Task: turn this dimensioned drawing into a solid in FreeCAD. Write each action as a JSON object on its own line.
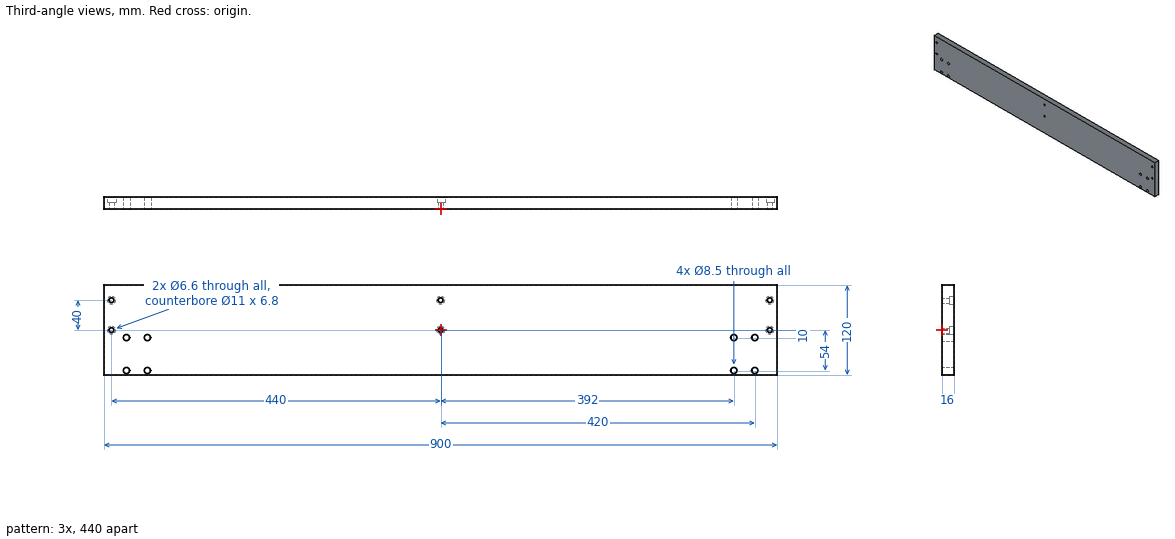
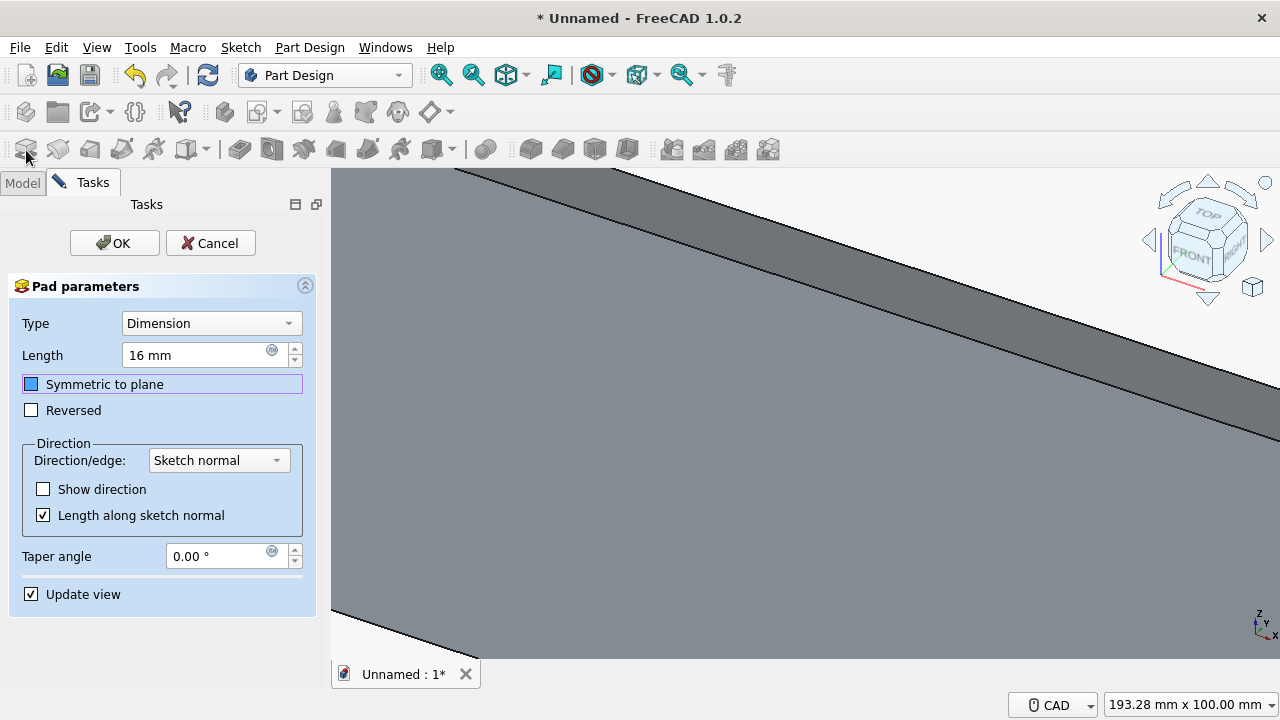
{"action": "left_click", "coordinate": [30, 410]}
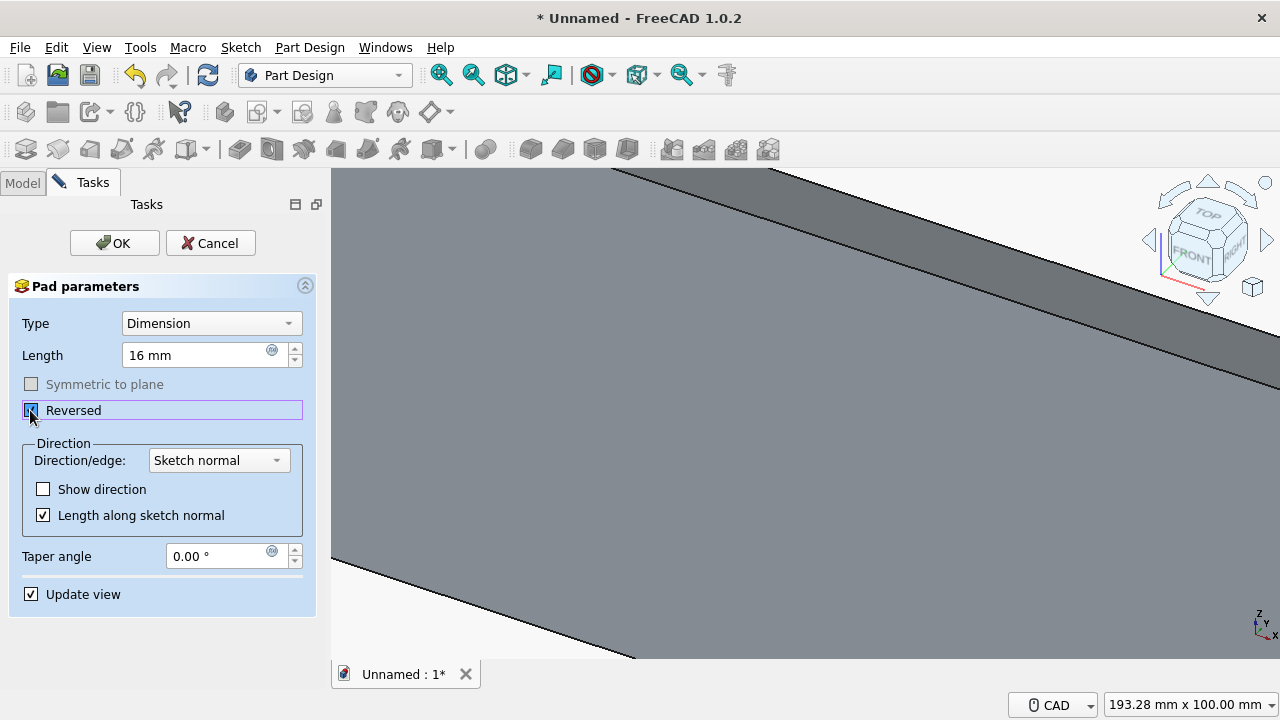
{"action": "left_click", "coordinate": [115, 243]}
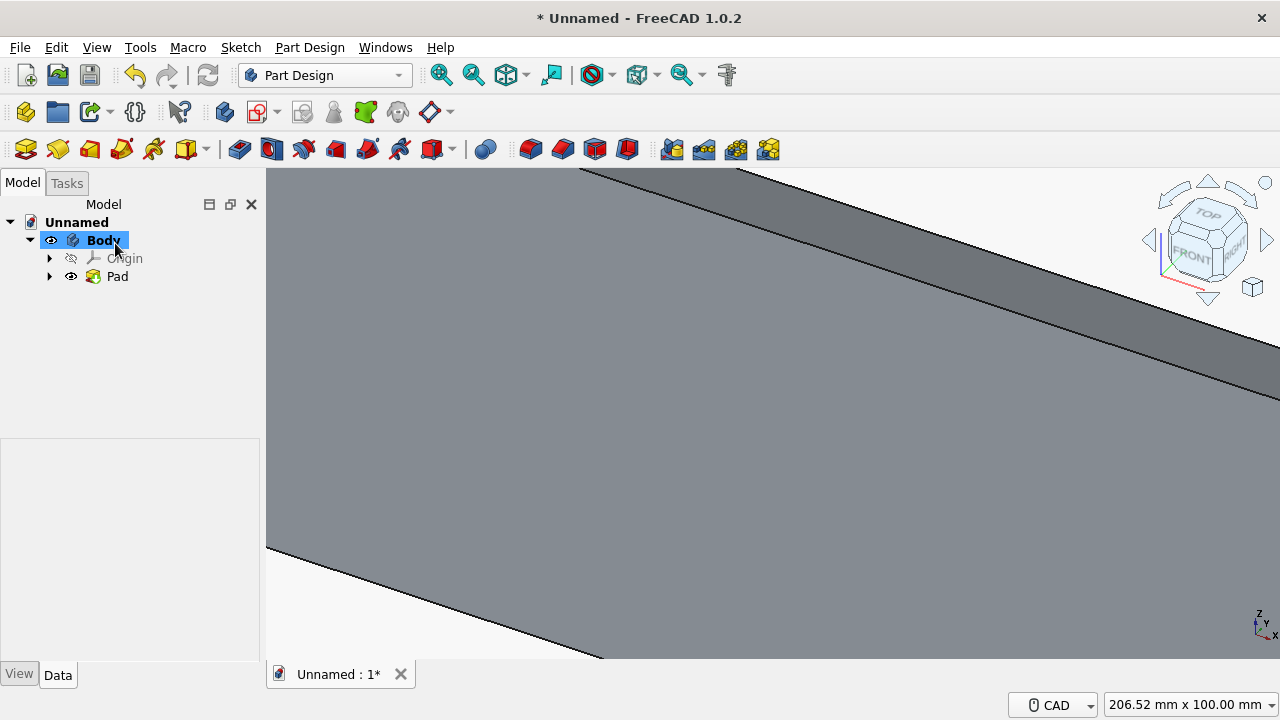
{"action": "key", "text": "v f"}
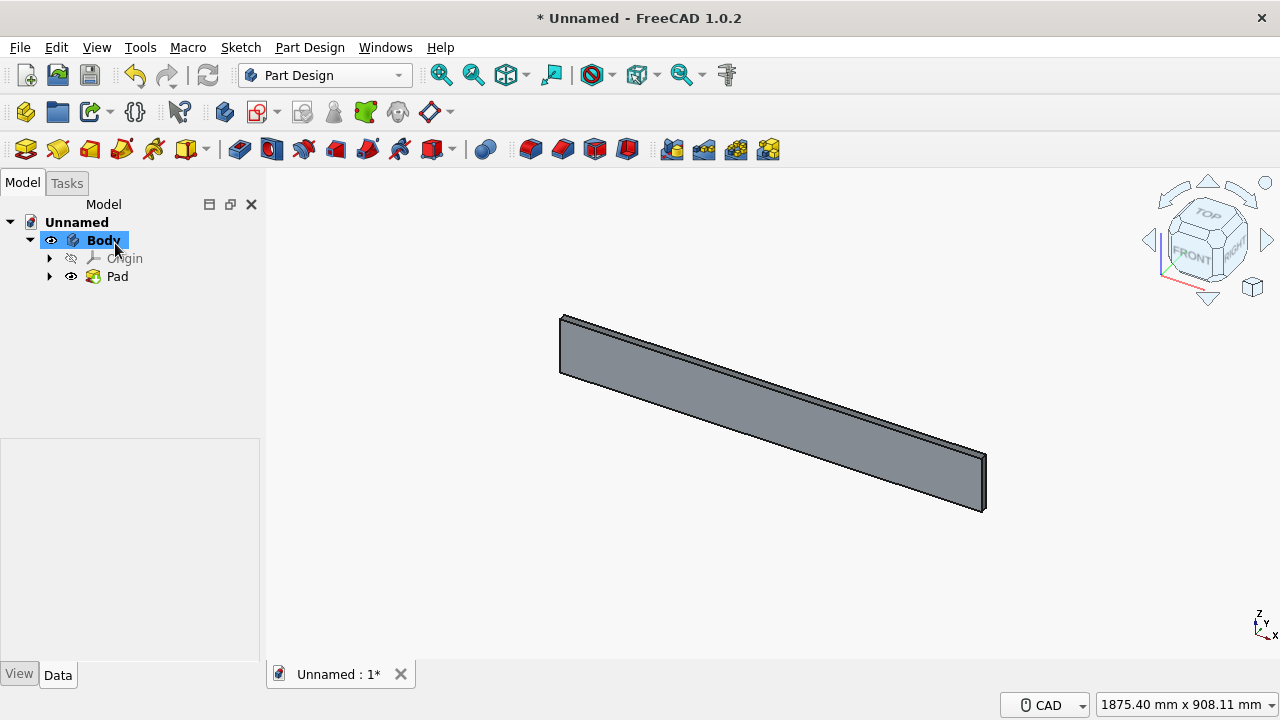
{"action": "key", "text": "4"}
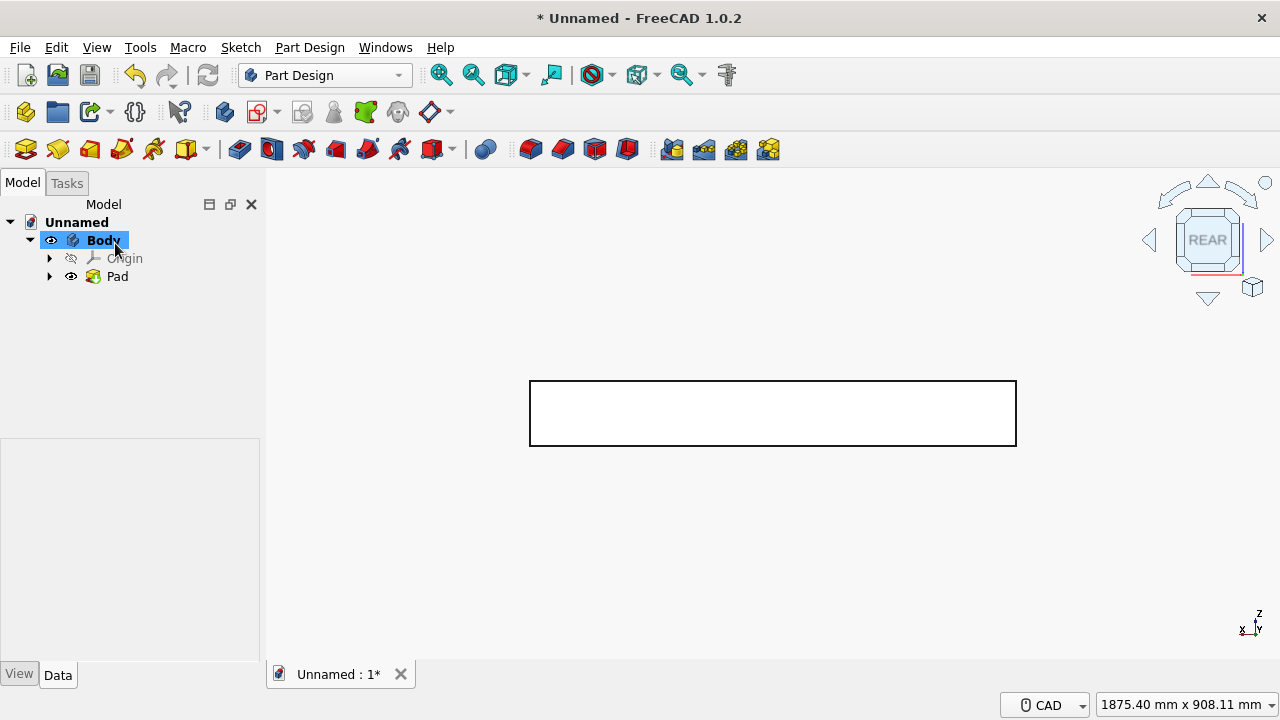
{"action": "left_click", "coordinate": [564, 413]}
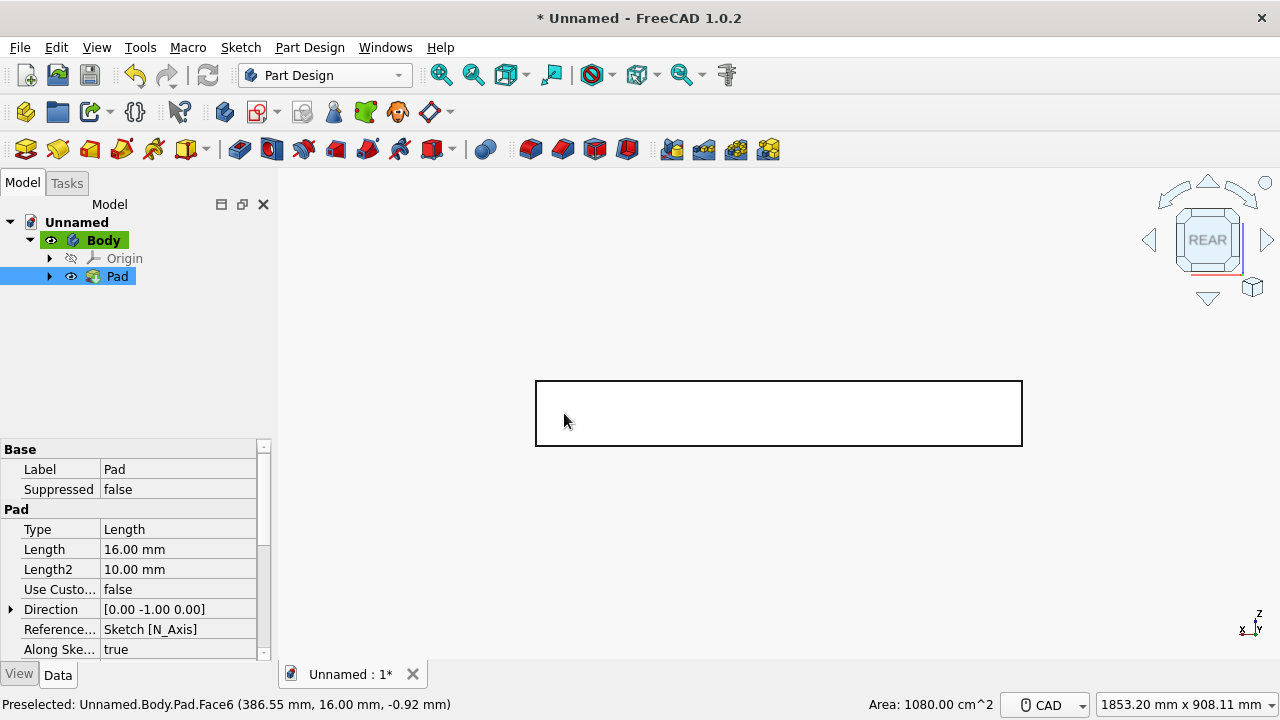
{"action": "left_click", "coordinate": [258, 112]}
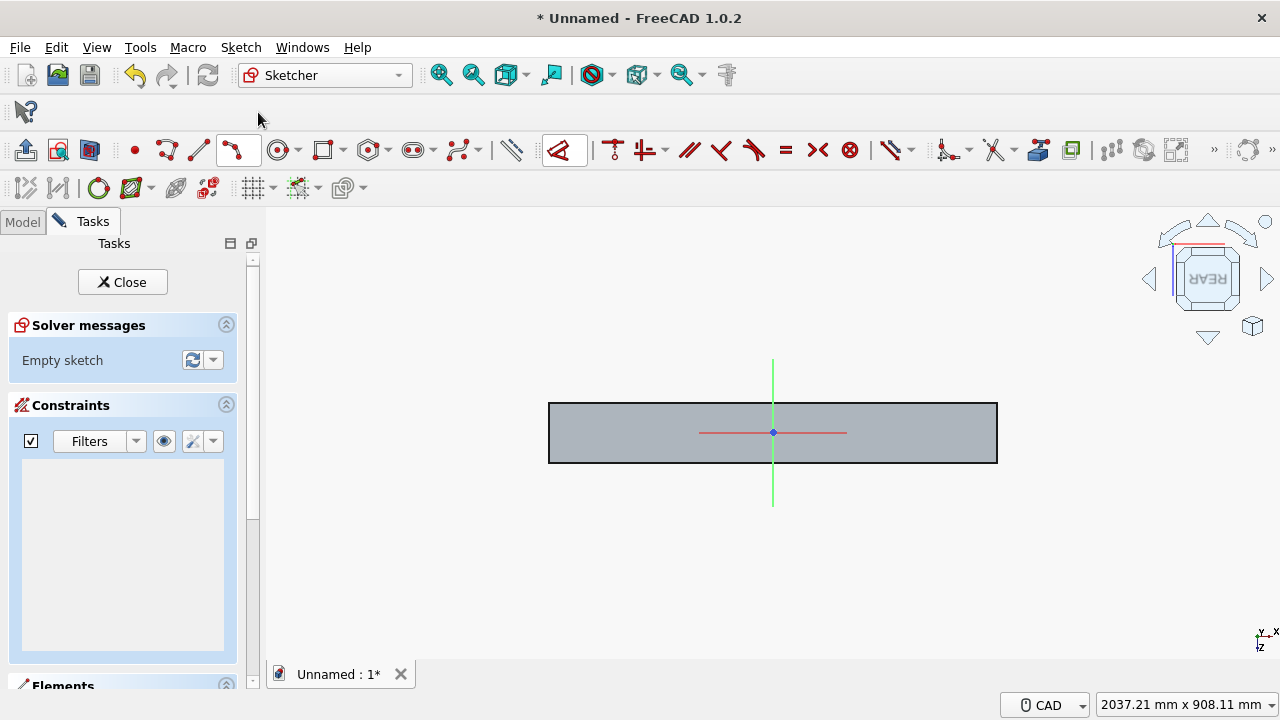
{"action": "scroll", "coordinate": [1002, 415], "scroll_direction": "up", "scroll_amount": 12}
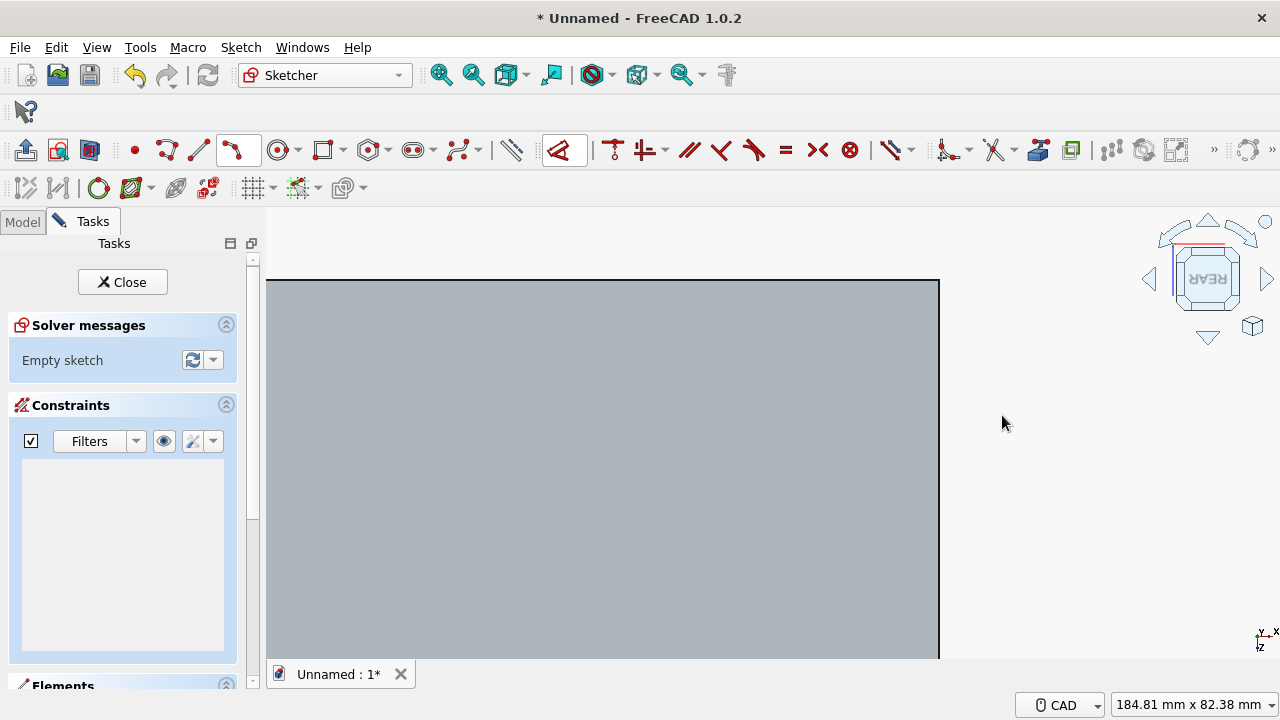
{"action": "left_click", "coordinate": [278, 150]}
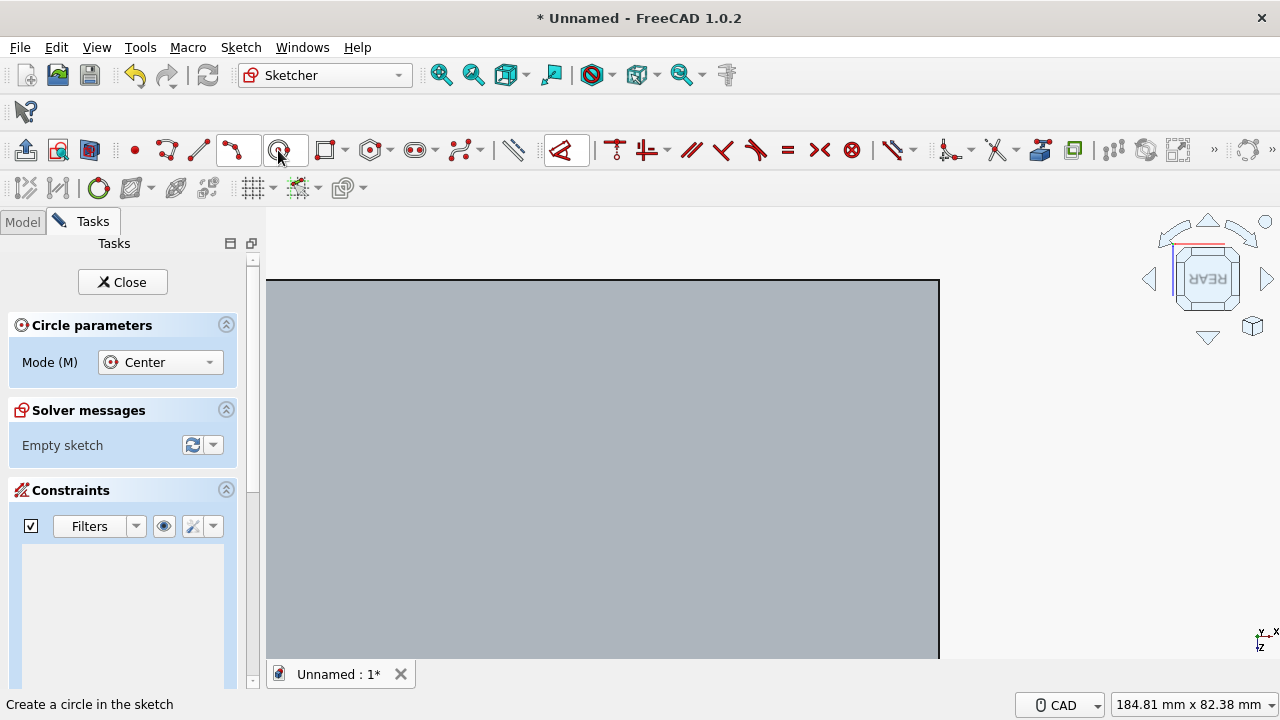
{"action": "left_click", "coordinate": [621, 313]}
{"action": "mouse_move", "coordinate": [638, 296]}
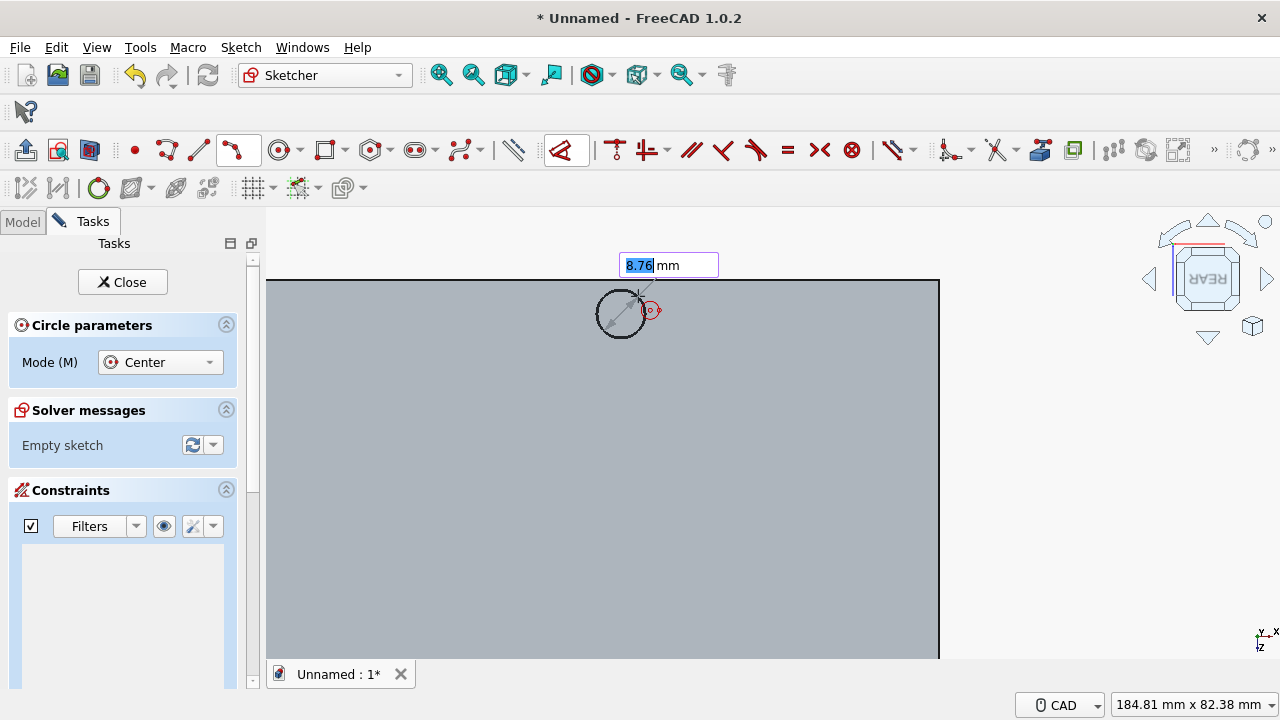
{"action": "type", "text": "8.5"}
{"action": "key", "text": "Return"}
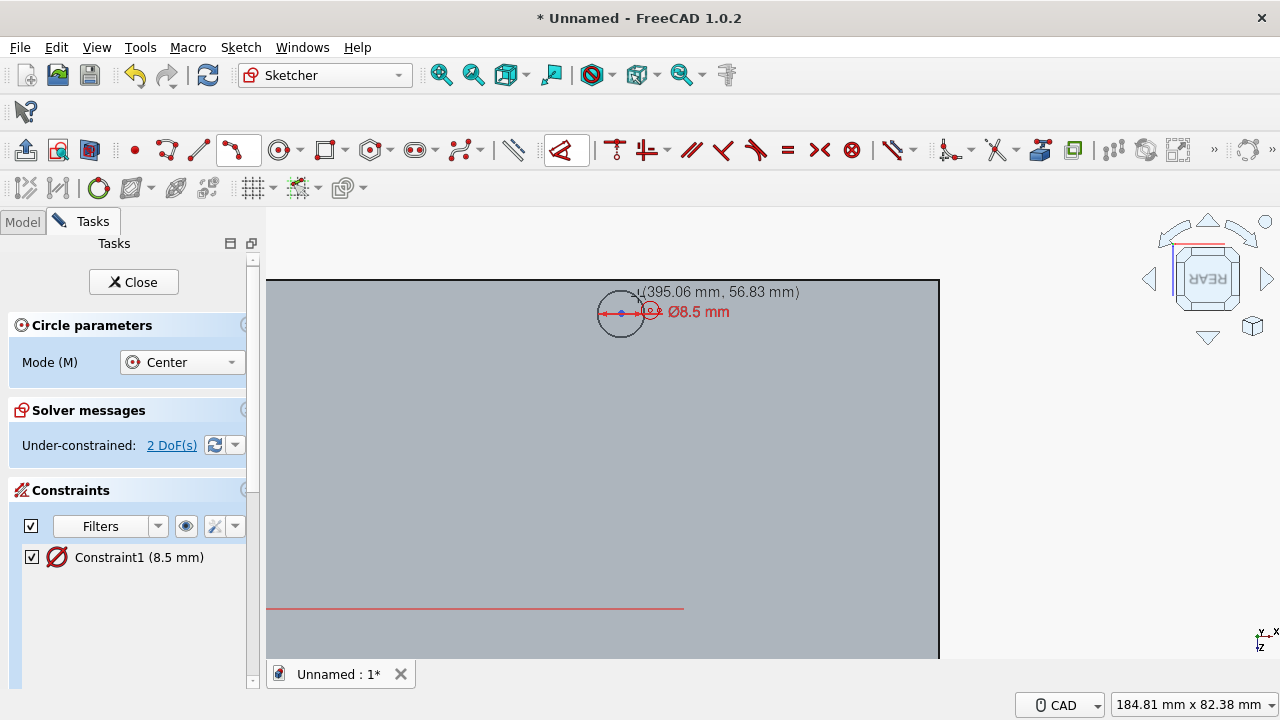
{"action": "left_click", "coordinate": [775, 313]}
{"action": "mouse_move", "coordinate": [791, 296]}